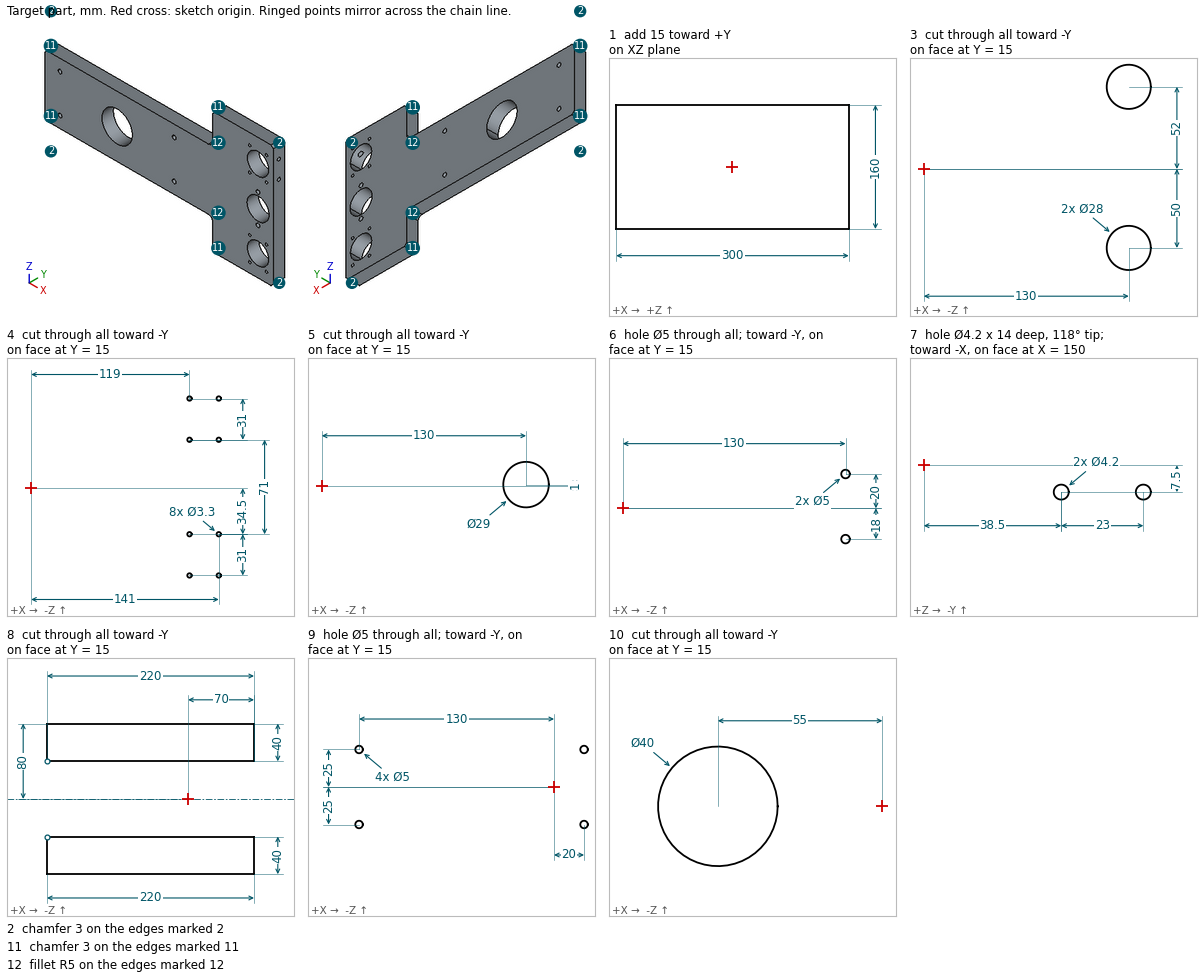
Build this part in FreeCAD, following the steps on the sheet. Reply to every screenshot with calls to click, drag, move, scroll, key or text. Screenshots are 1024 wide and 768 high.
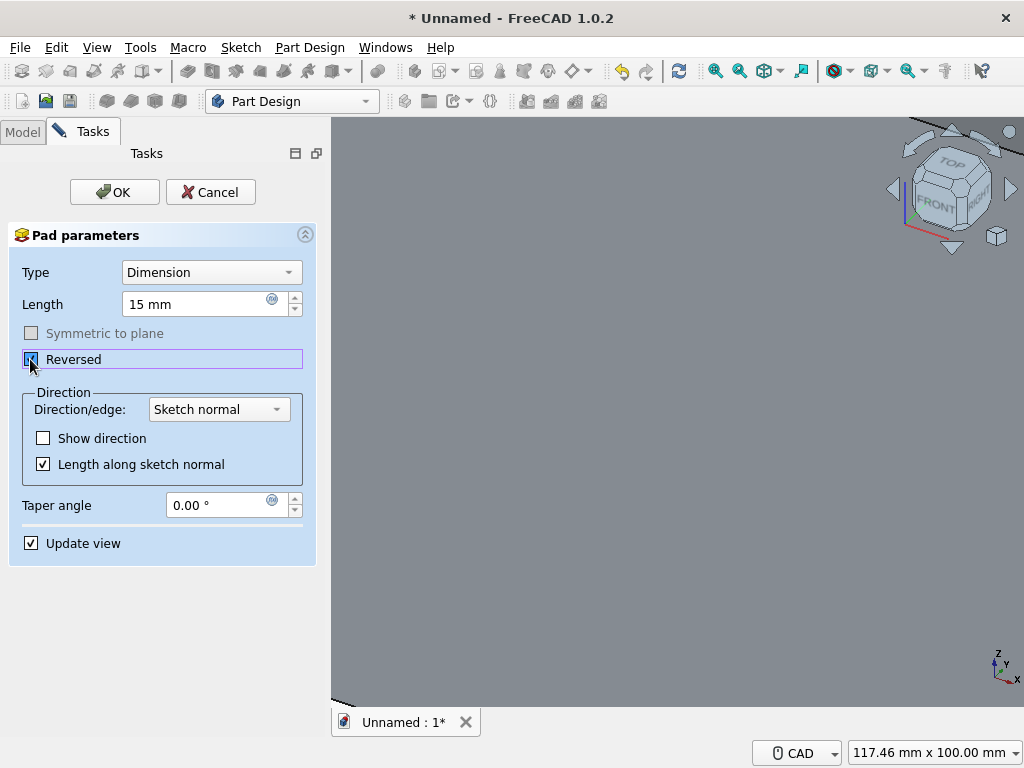
click(115, 192)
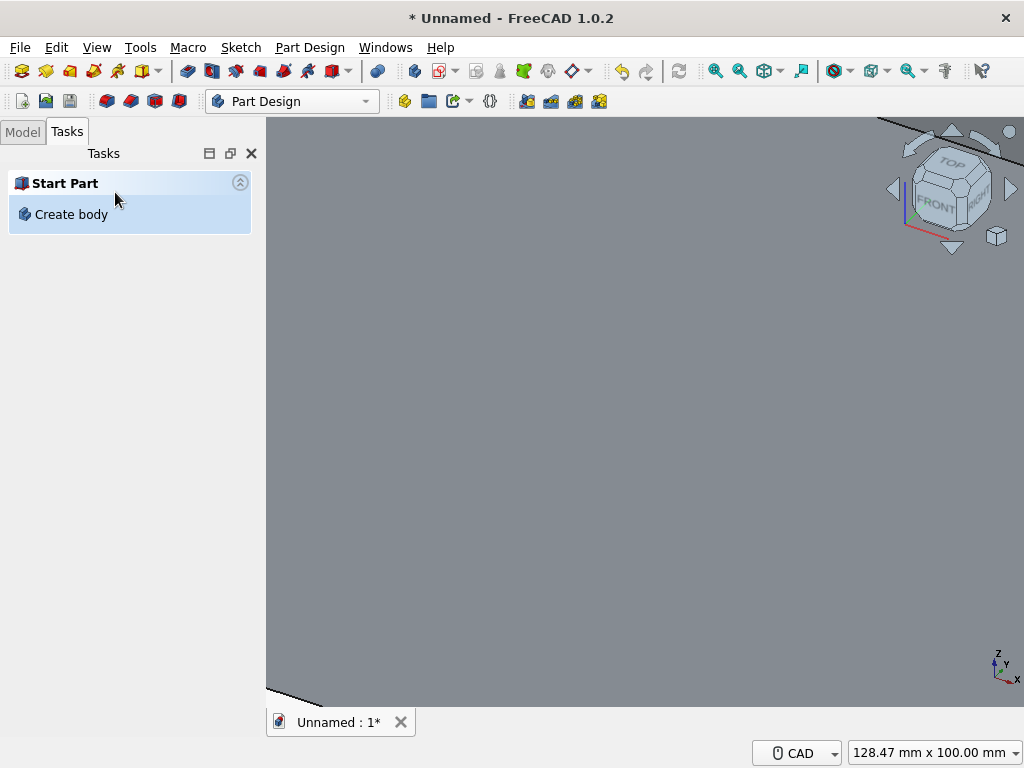
click(716, 72)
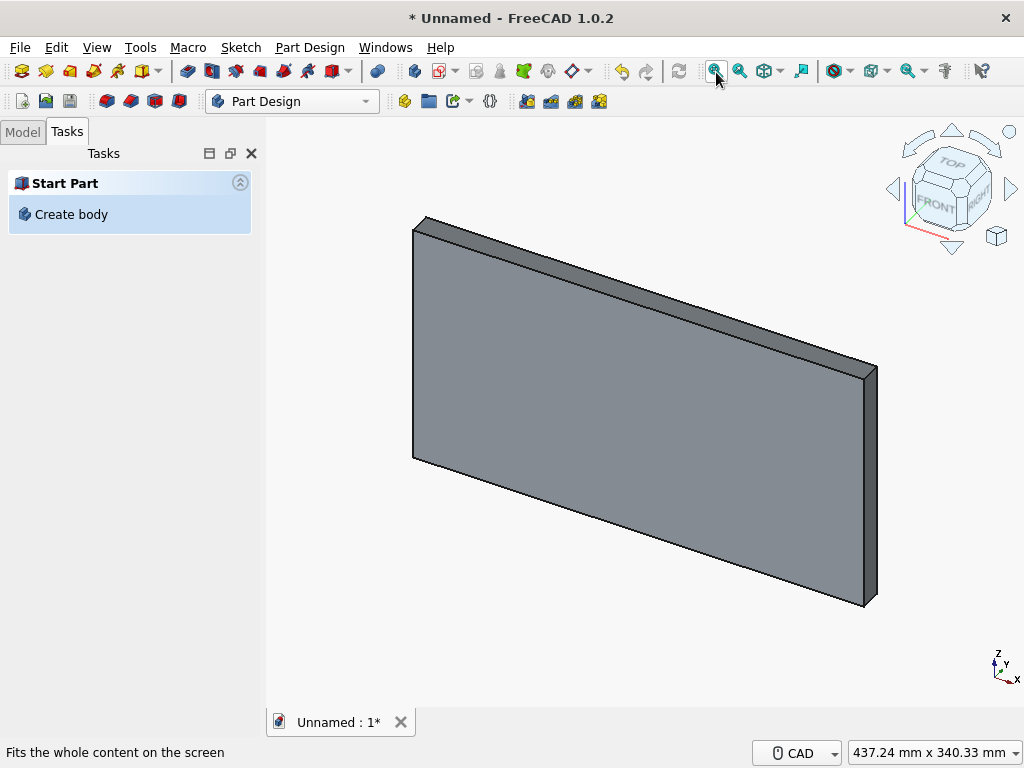
click(870, 372)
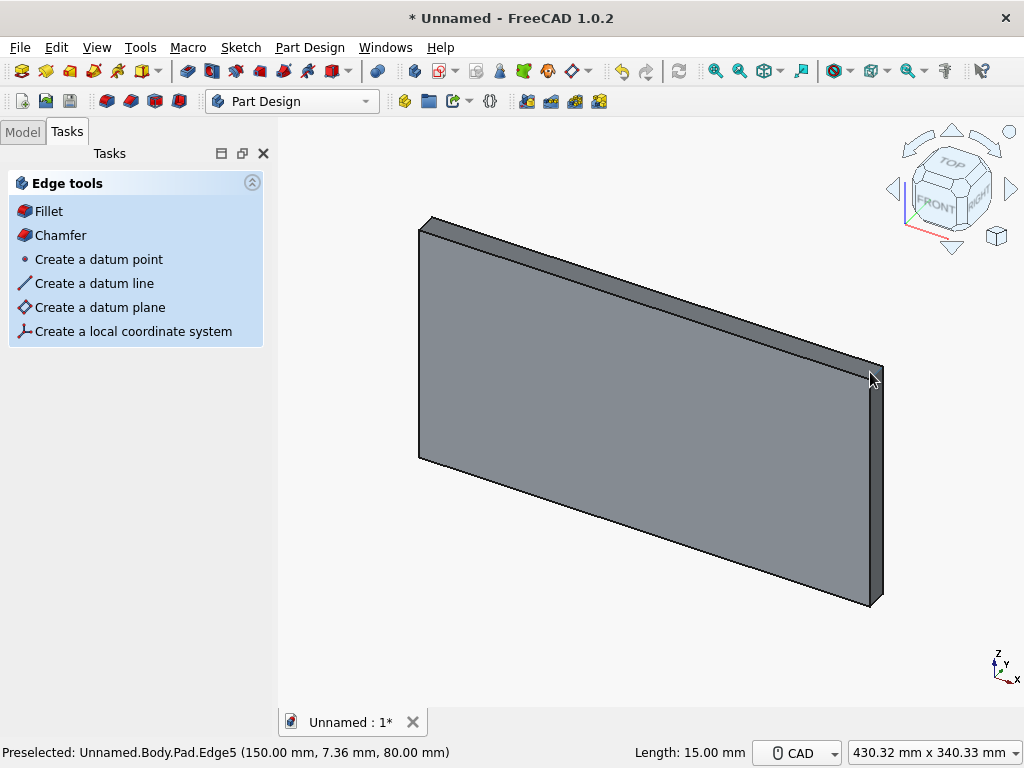
key(0)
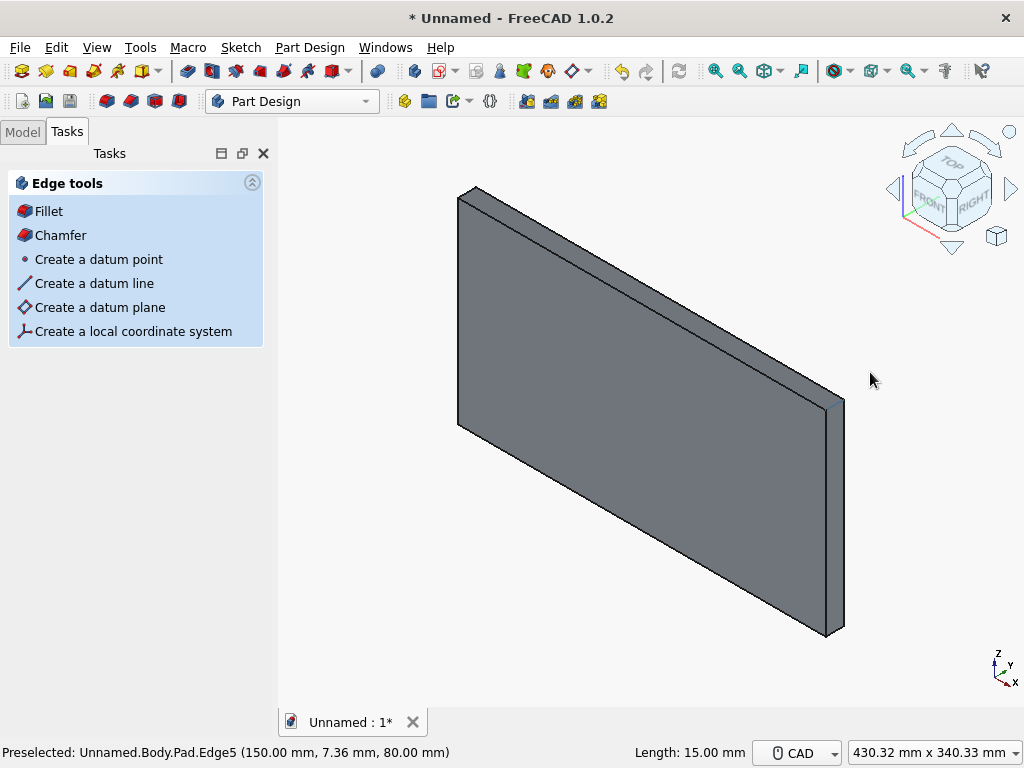
key(2)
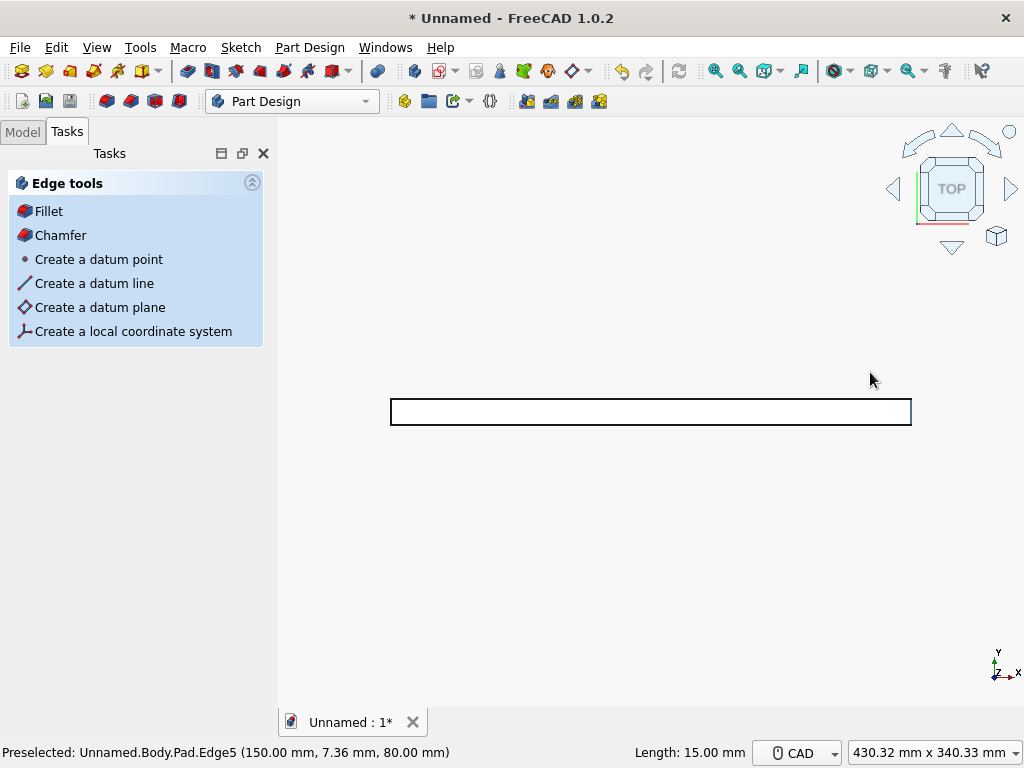
click(391, 411, ctrl)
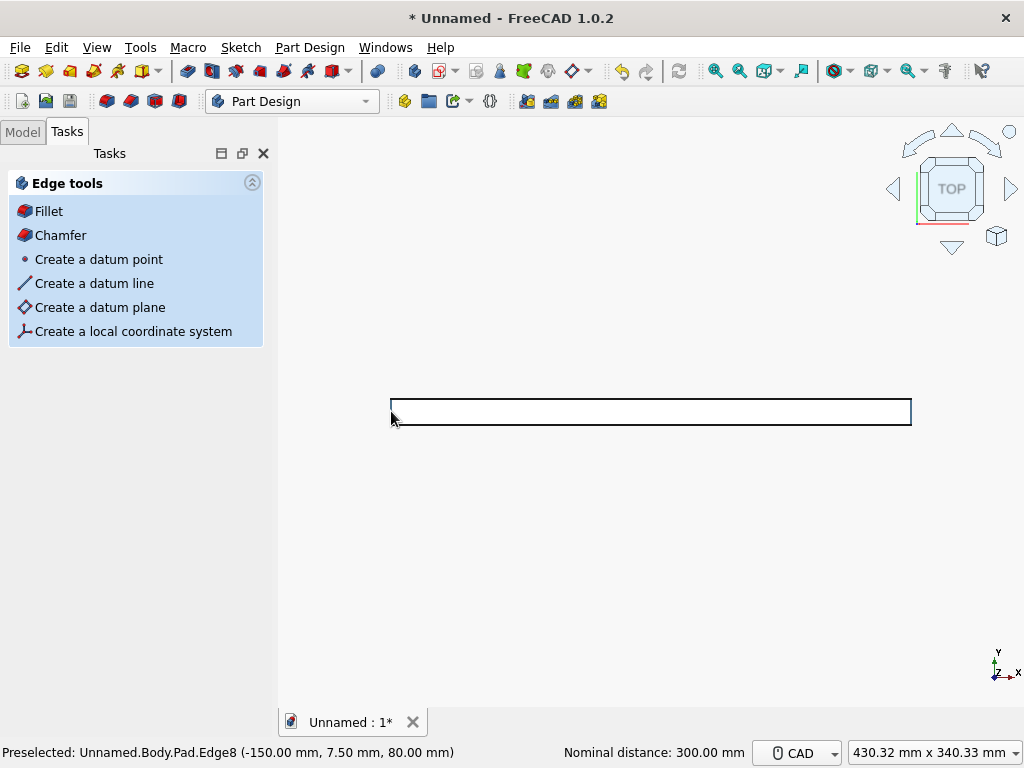
key(1)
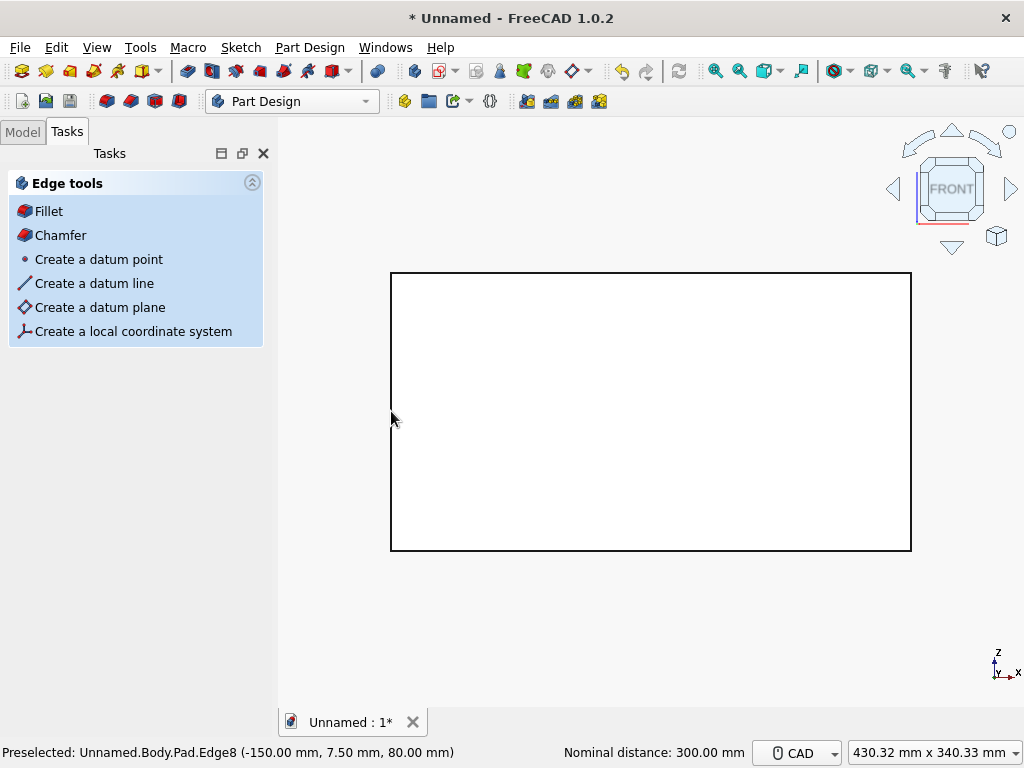
key(3)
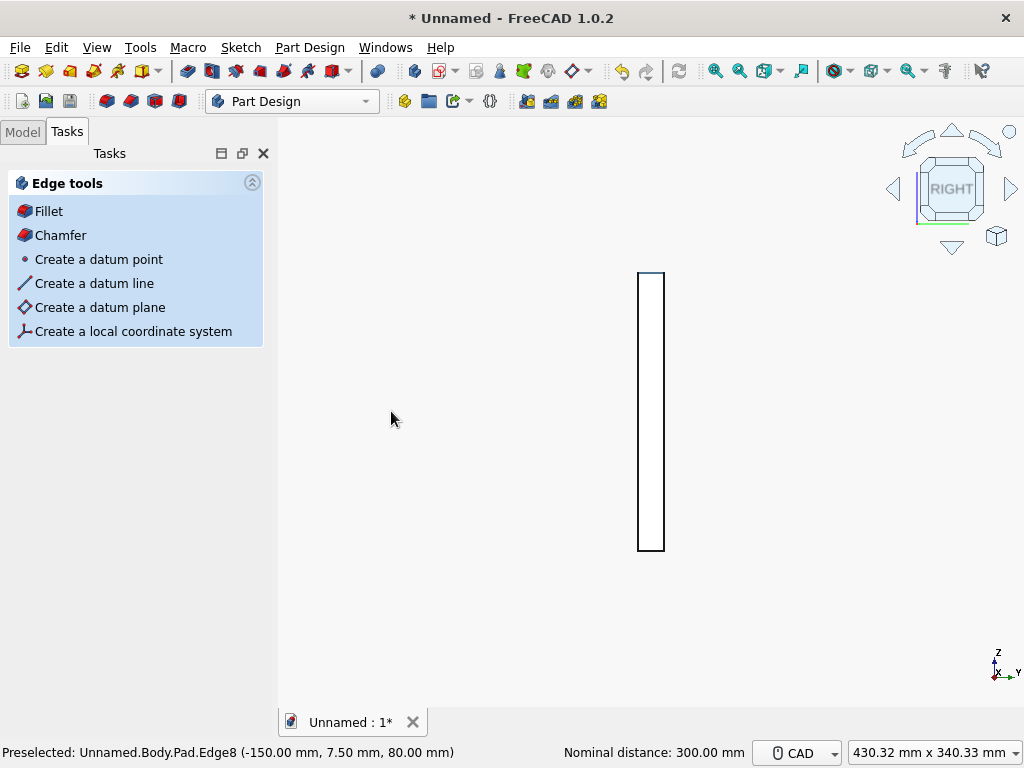
click(651, 550, ctrl)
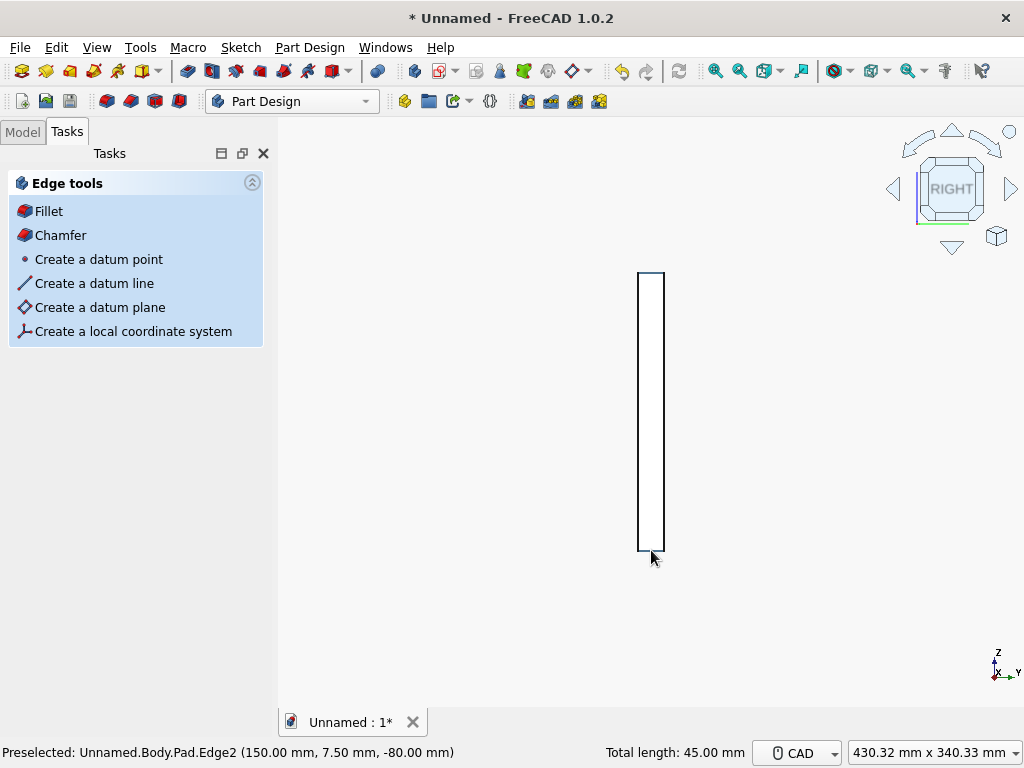
key(5)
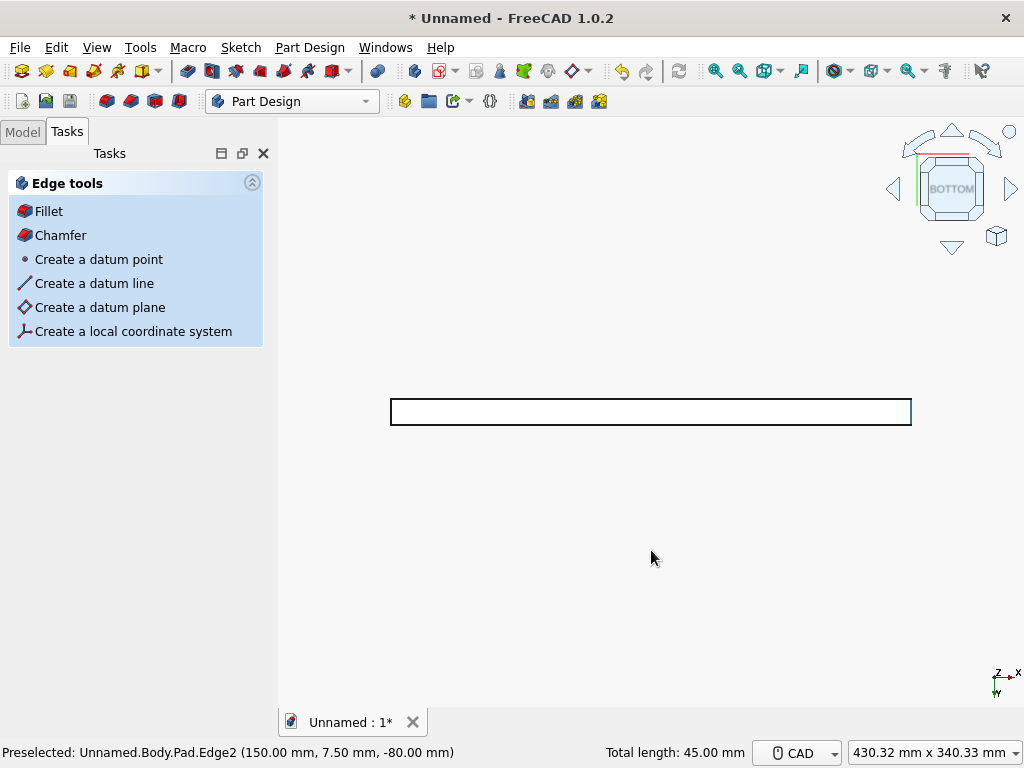
click(391, 411, ctrl)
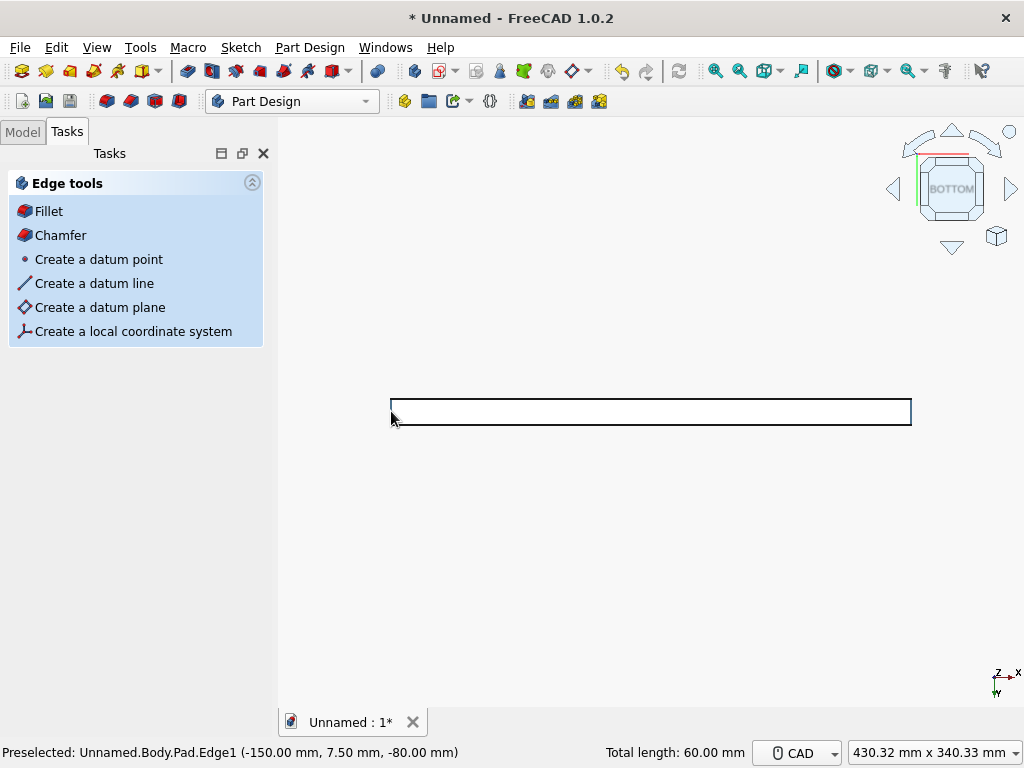
click(132, 102)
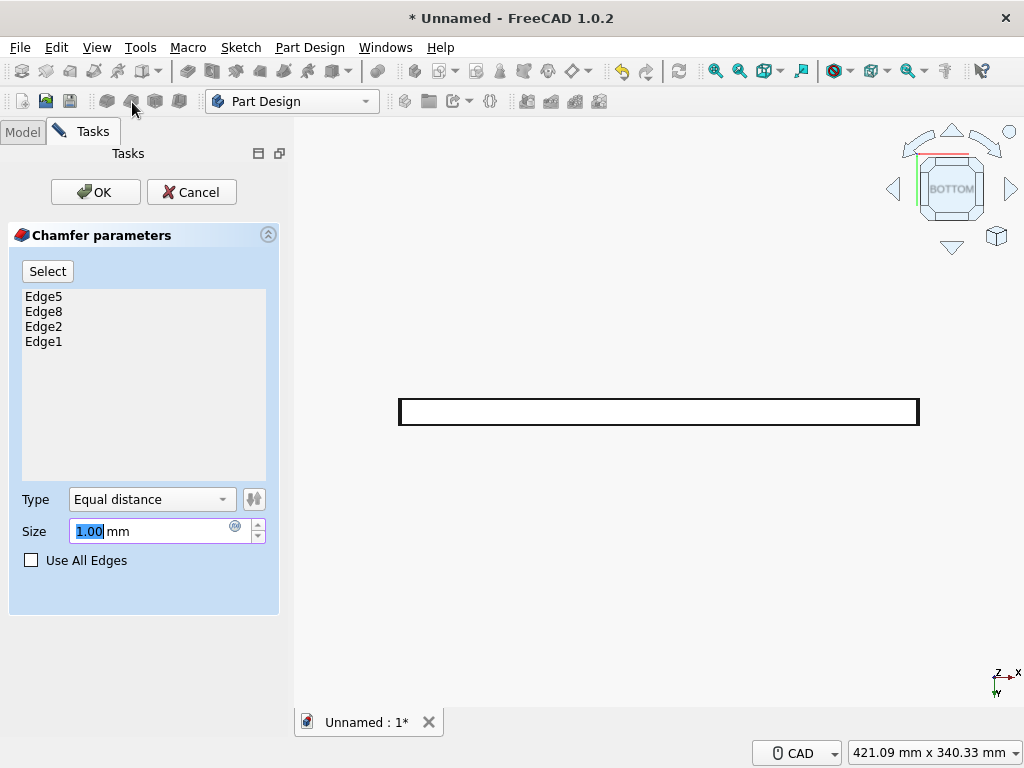
text(3)
key(Tab)